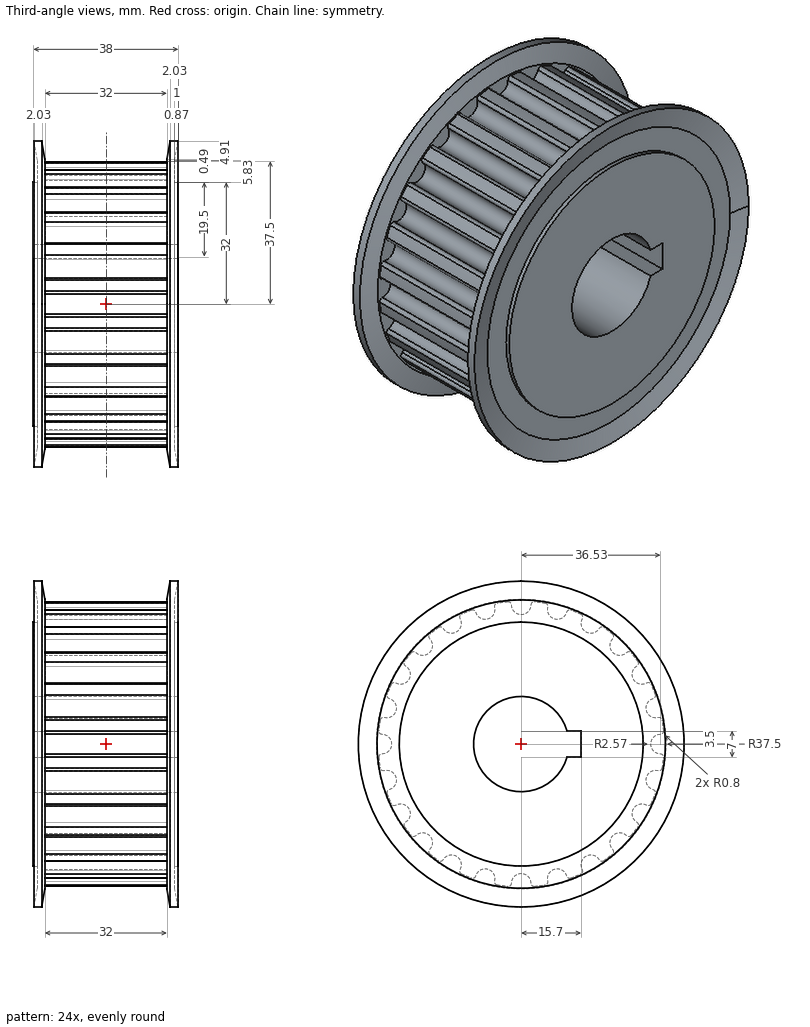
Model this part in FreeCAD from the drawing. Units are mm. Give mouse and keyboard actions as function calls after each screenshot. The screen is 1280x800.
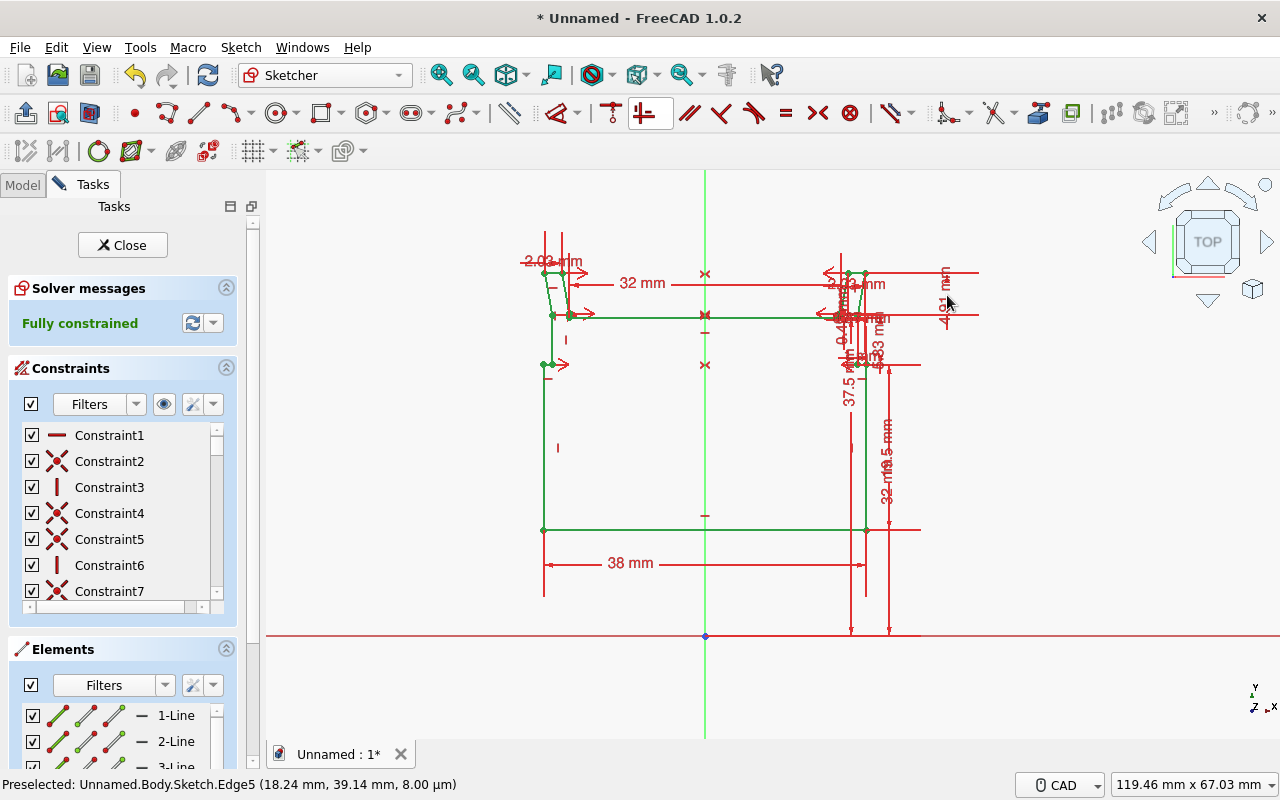
click(123, 245)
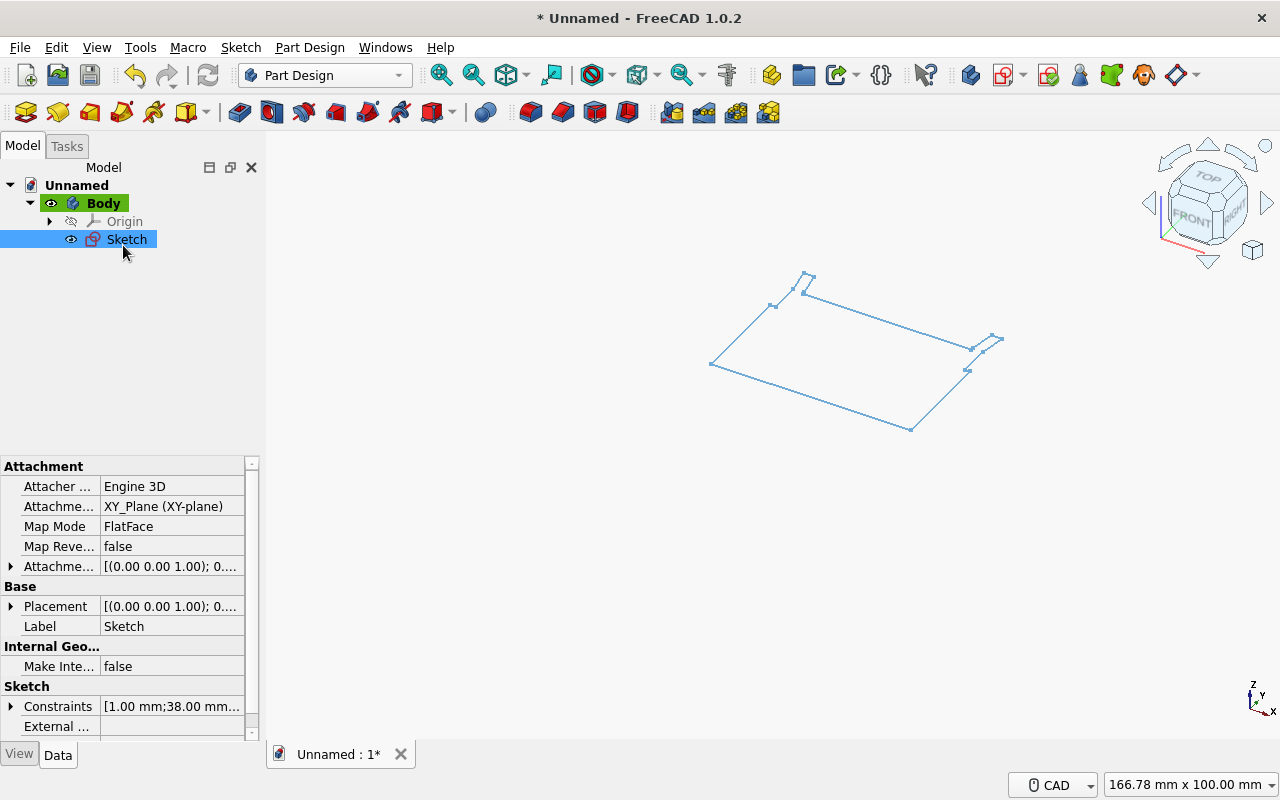
click(58, 112)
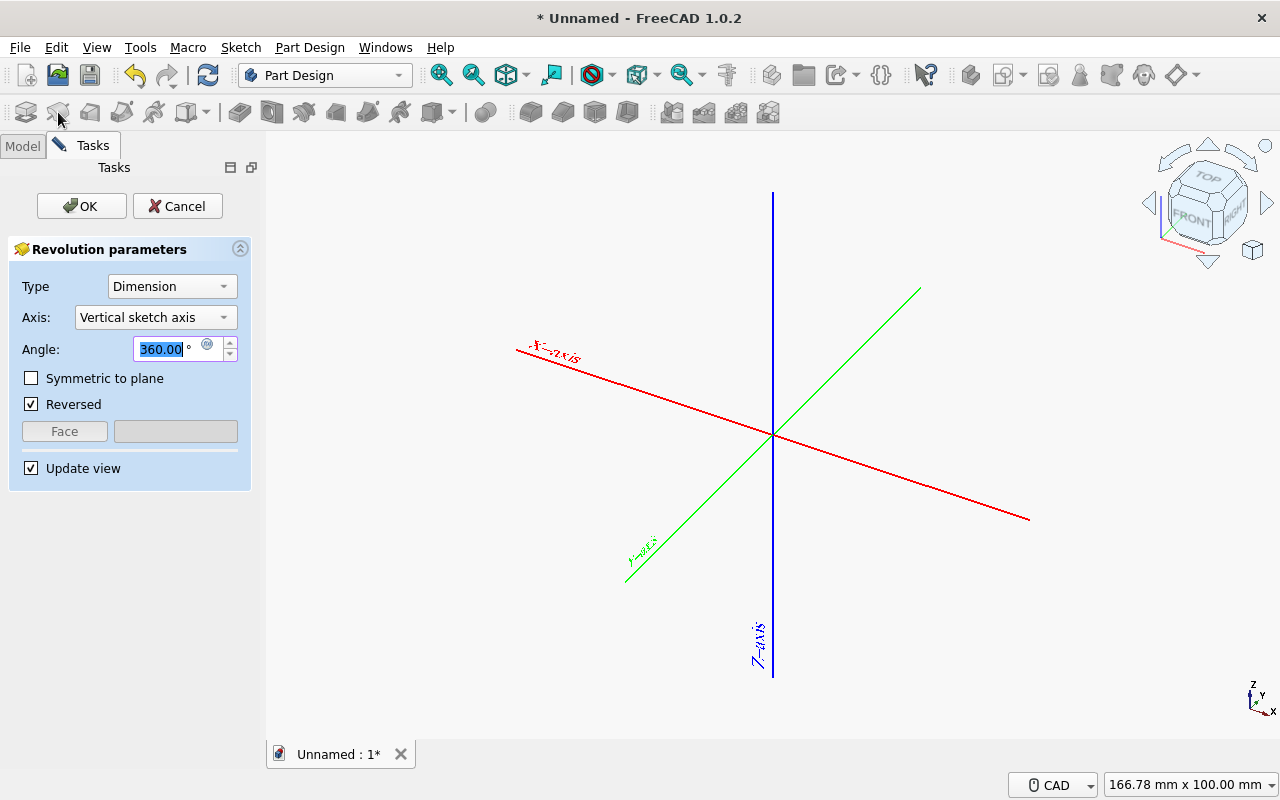
click(156, 318)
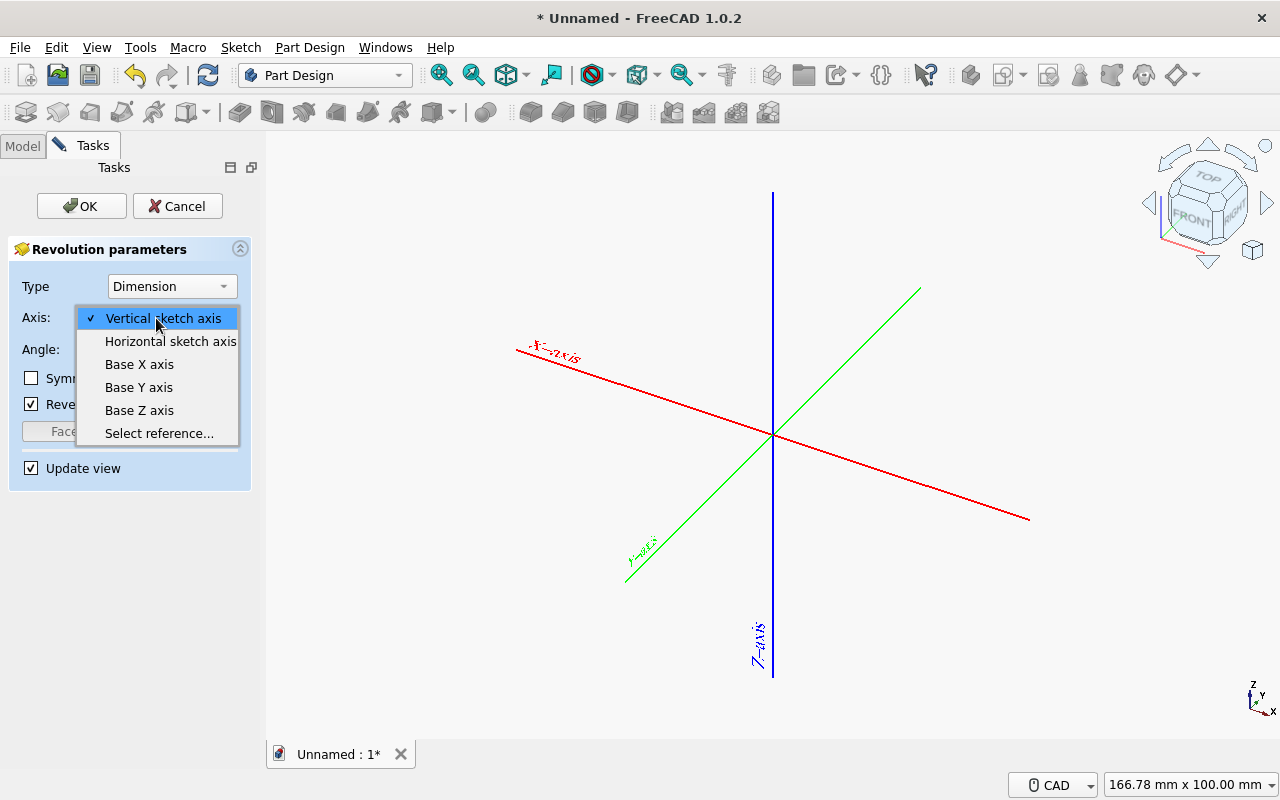
click(156, 342)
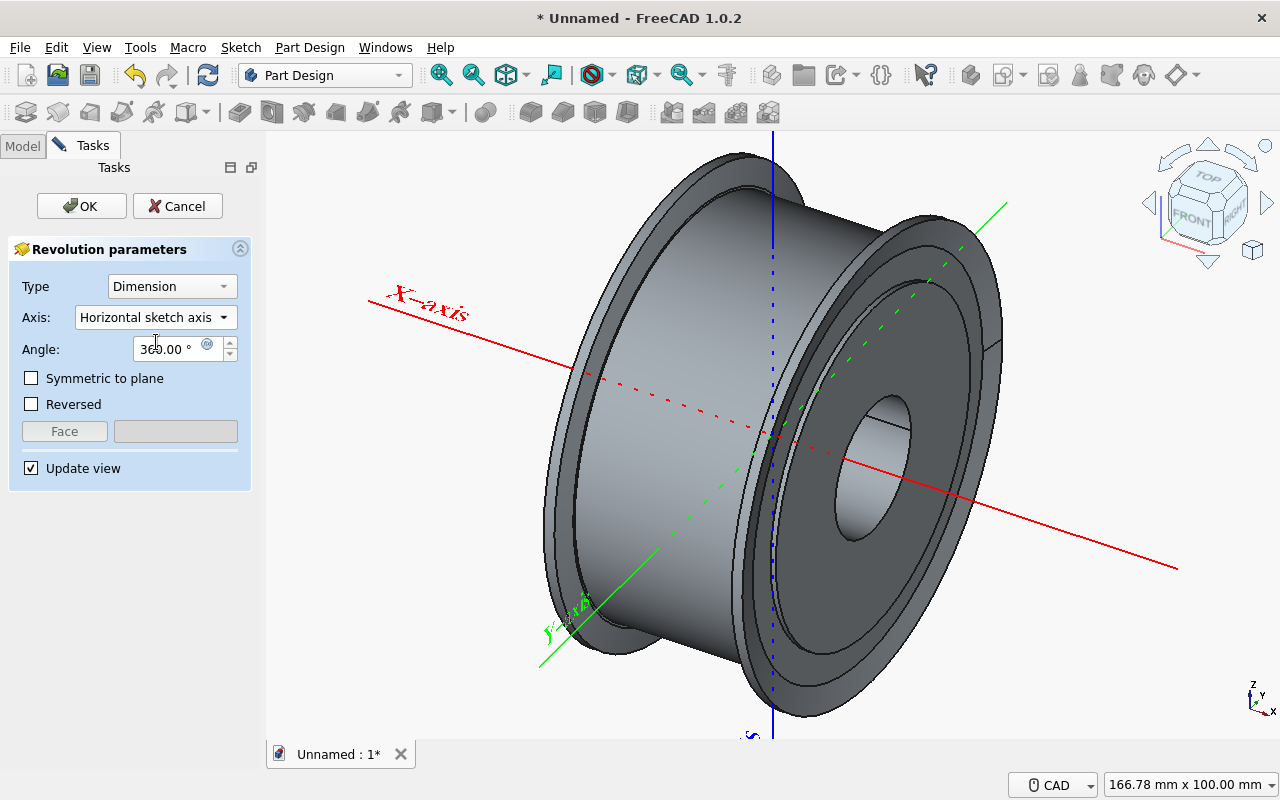
click(82, 206)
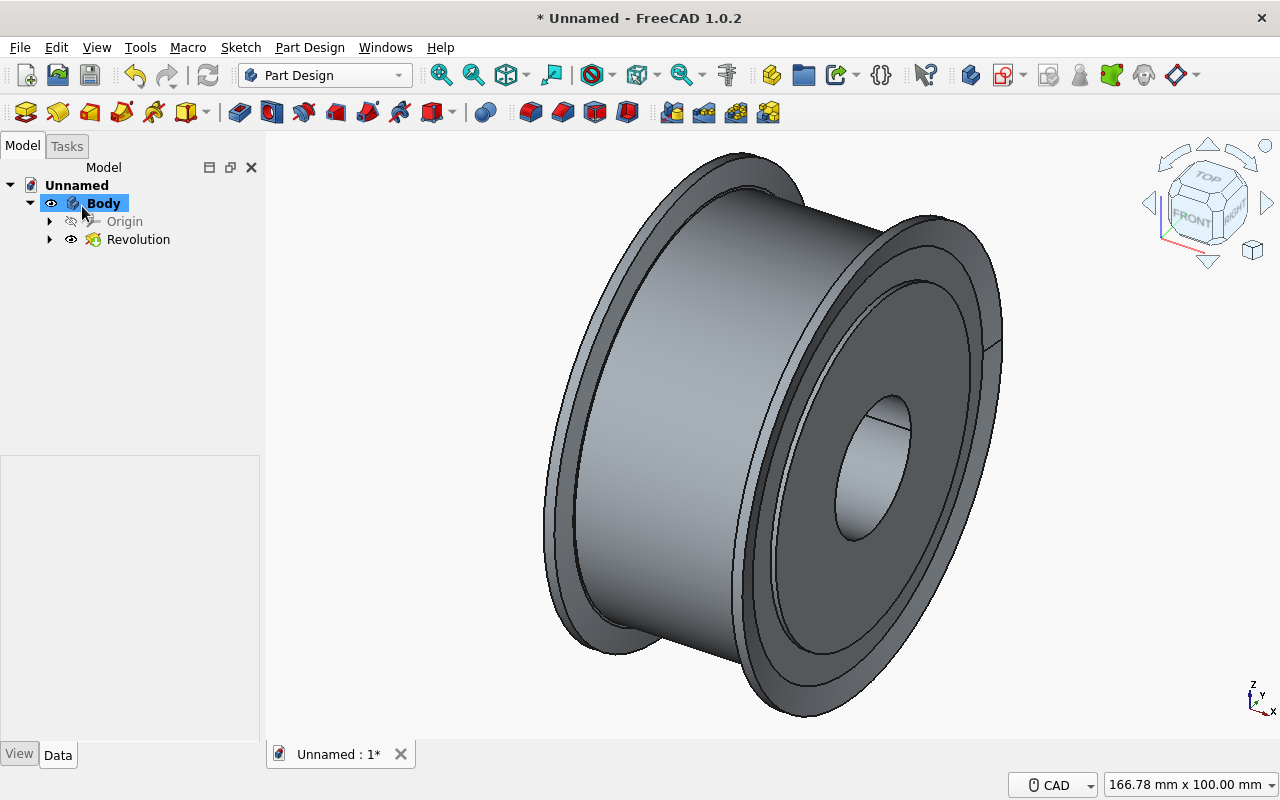
click(442, 76)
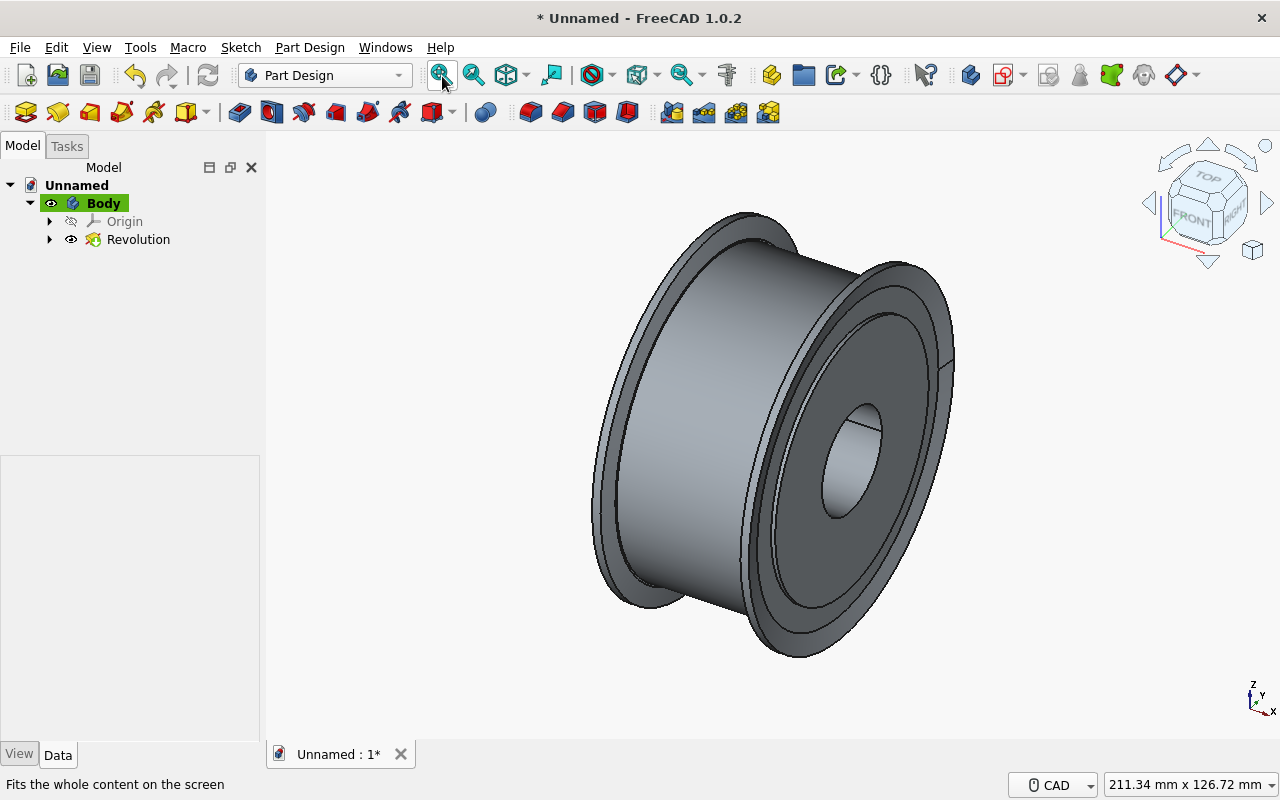
click(896, 381)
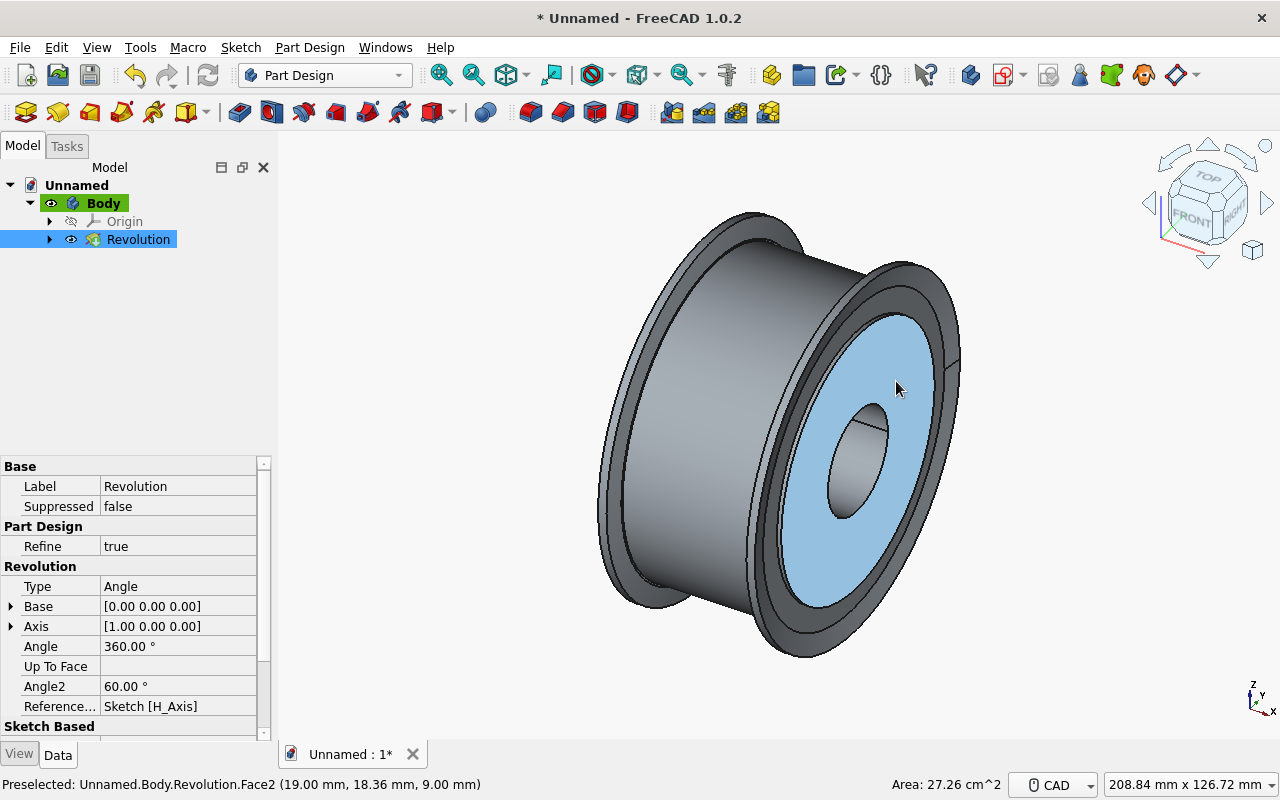
click(1004, 76)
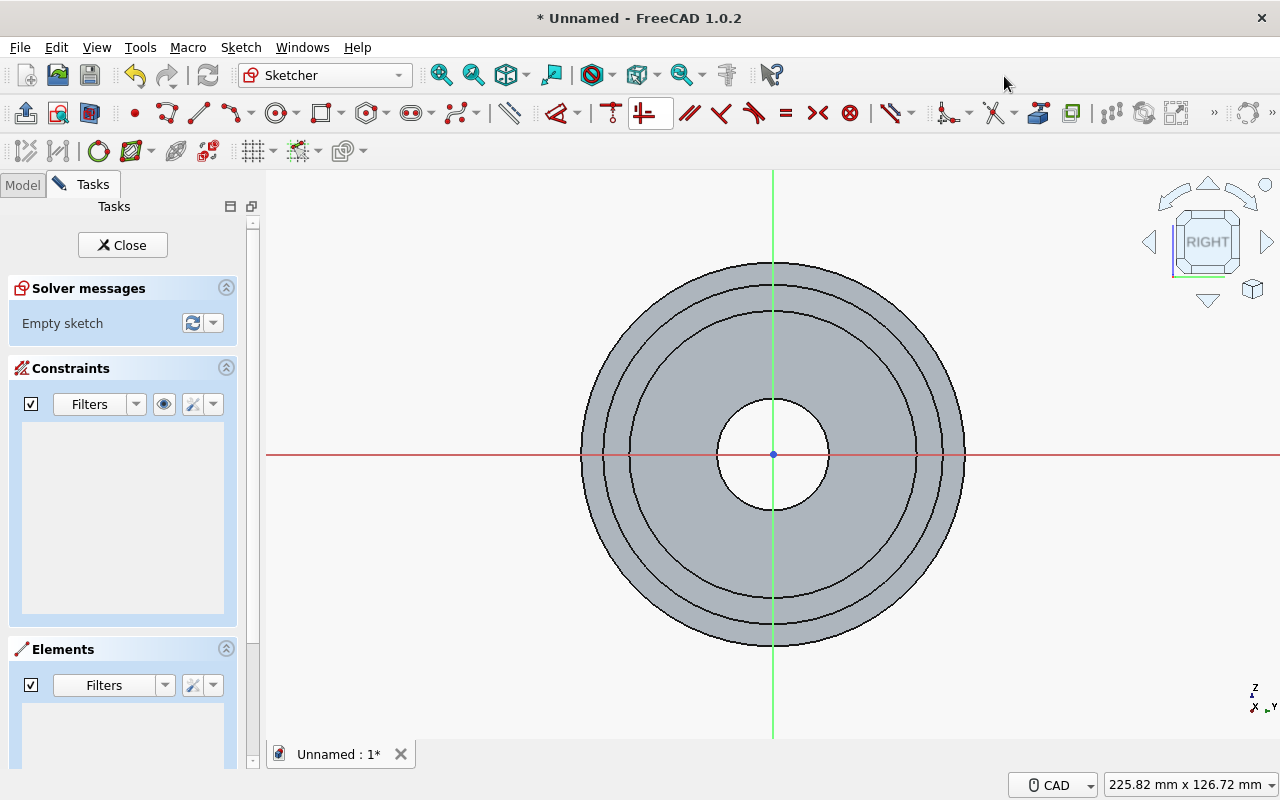
scroll(821, 454, up, 11)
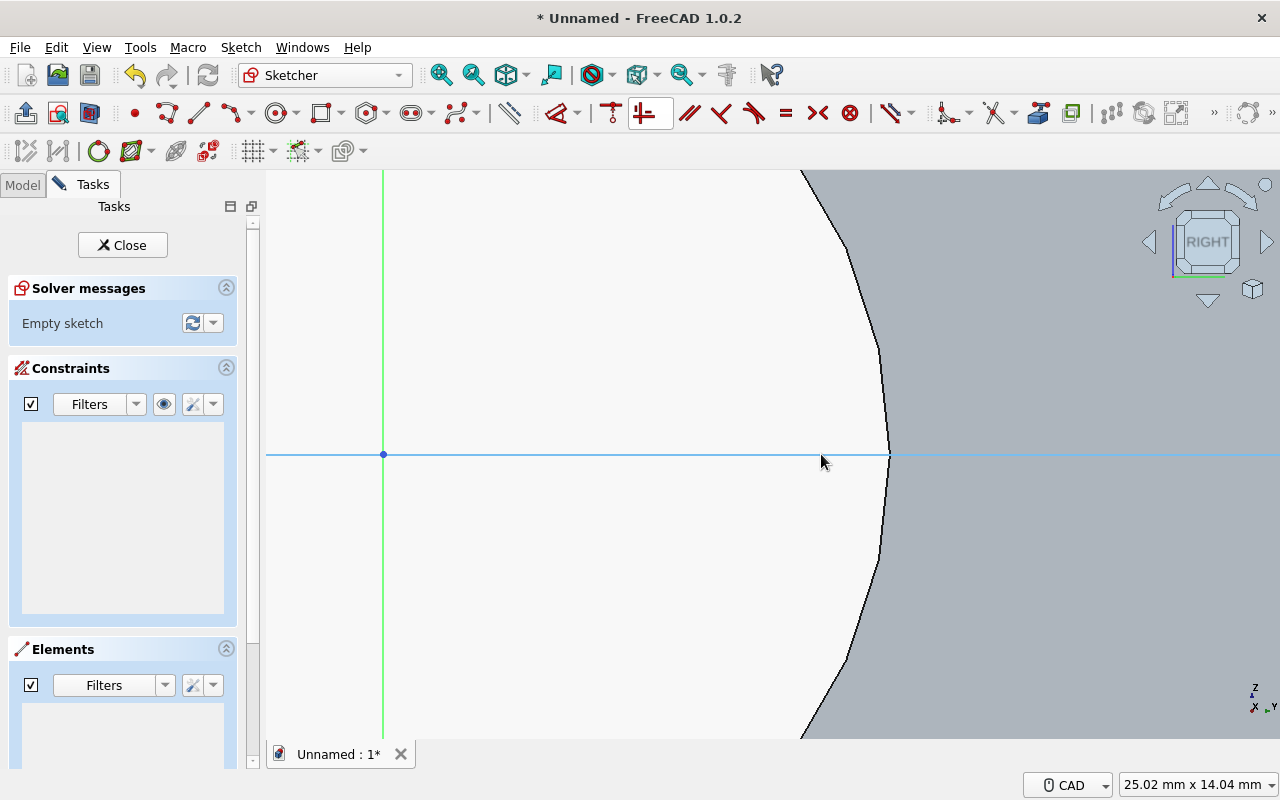
click(322, 114)